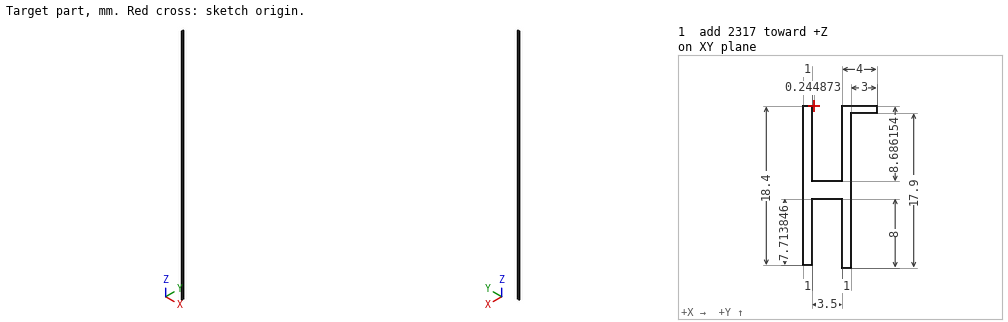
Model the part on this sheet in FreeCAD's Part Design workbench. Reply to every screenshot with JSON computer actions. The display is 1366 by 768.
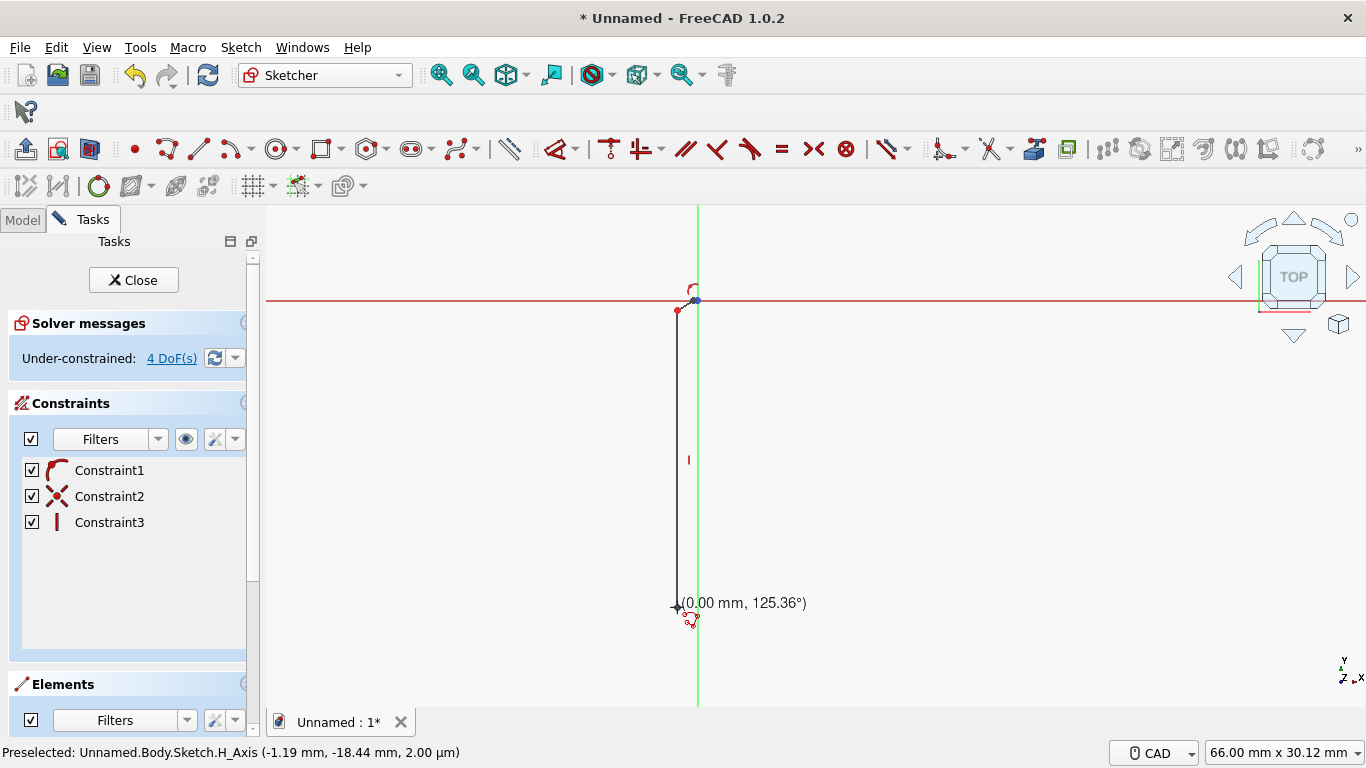
{"action": "scroll", "coordinate": [694, 607], "scroll_direction": "up", "scroll_amount": 7}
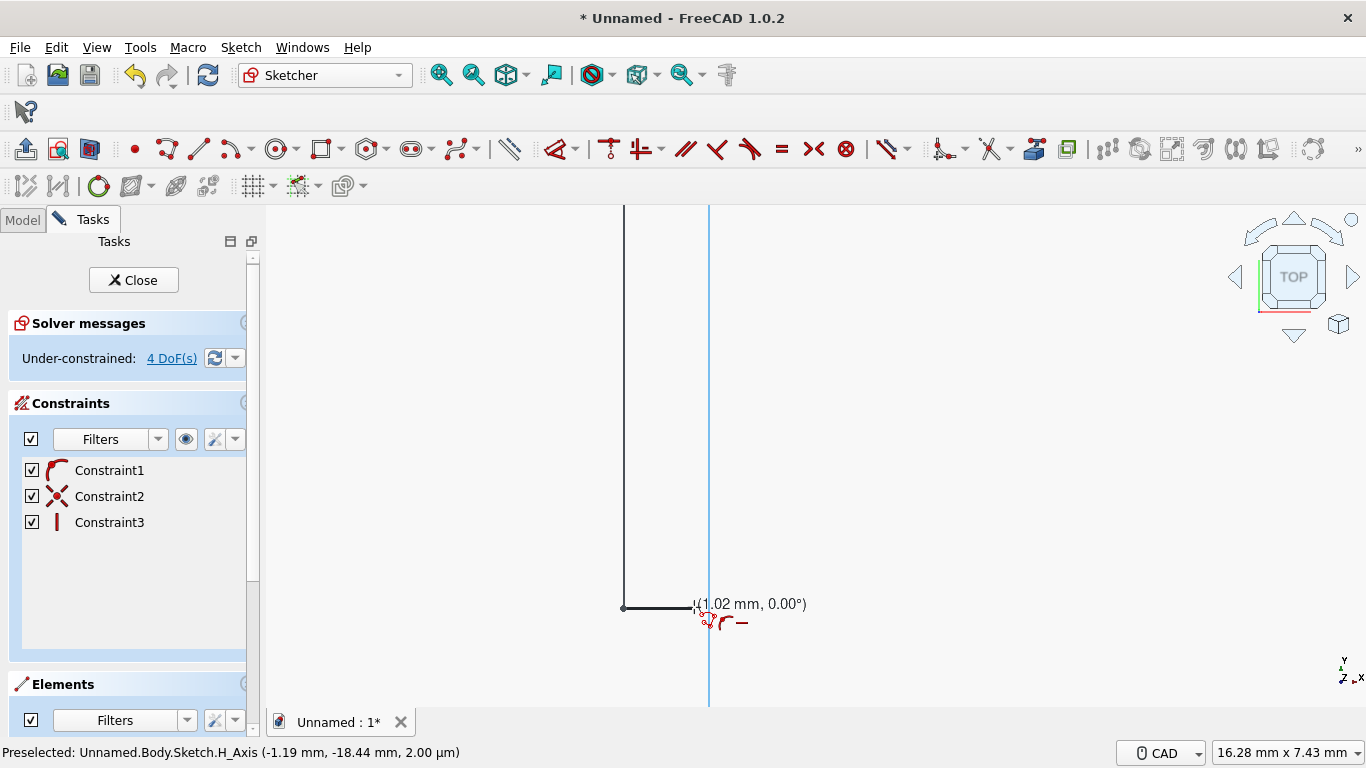
{"action": "left_click", "coordinate": [692, 605]}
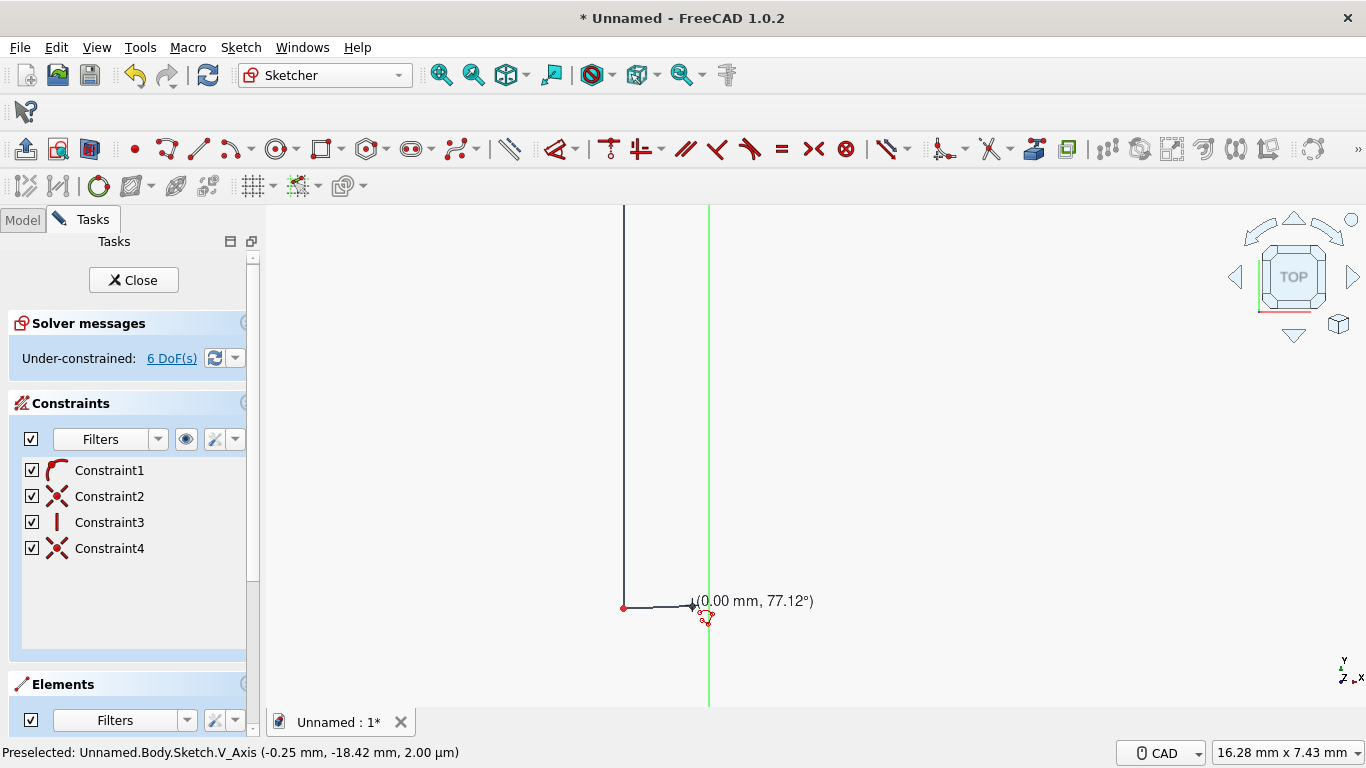
{"action": "scroll", "coordinate": [694, 607], "scroll_direction": "down", "scroll_amount": 7}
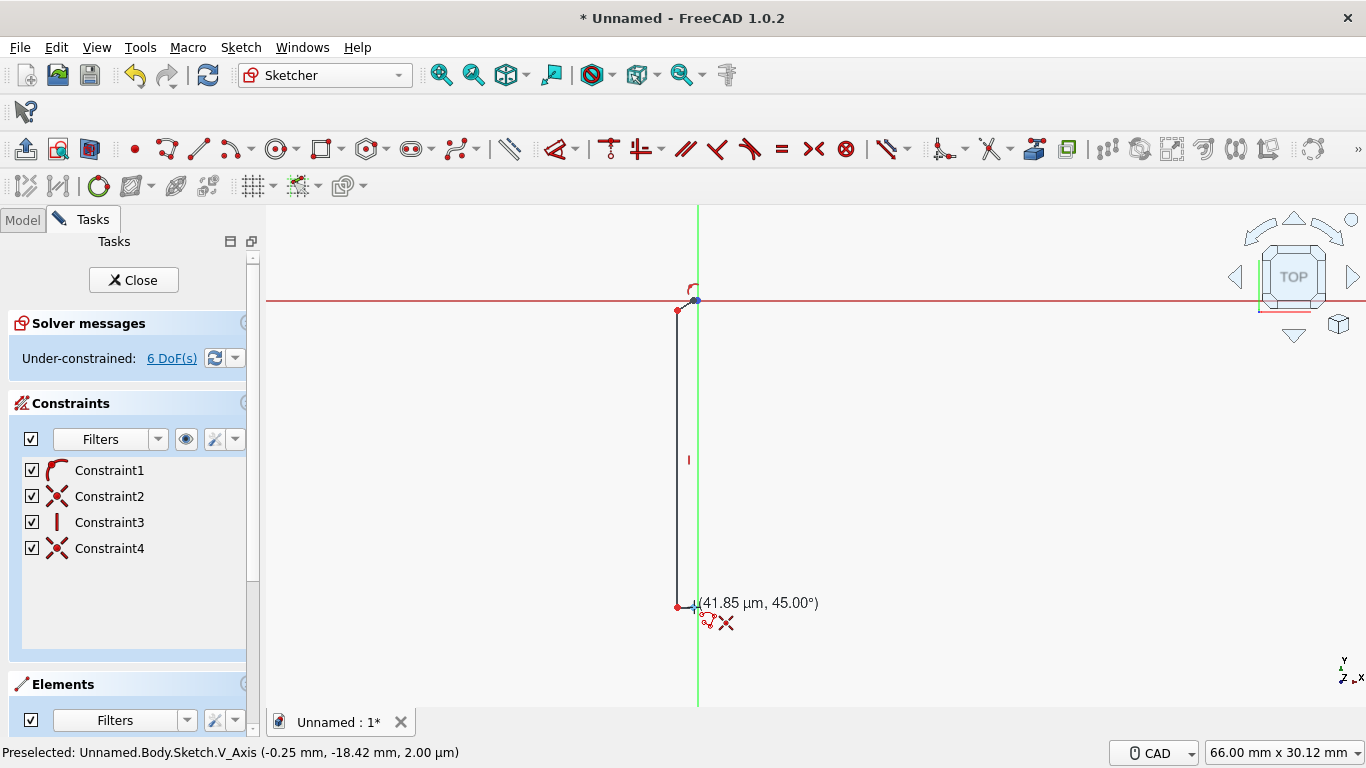
{"action": "scroll", "coordinate": [694, 479], "scroll_direction": "up", "scroll_amount": 7}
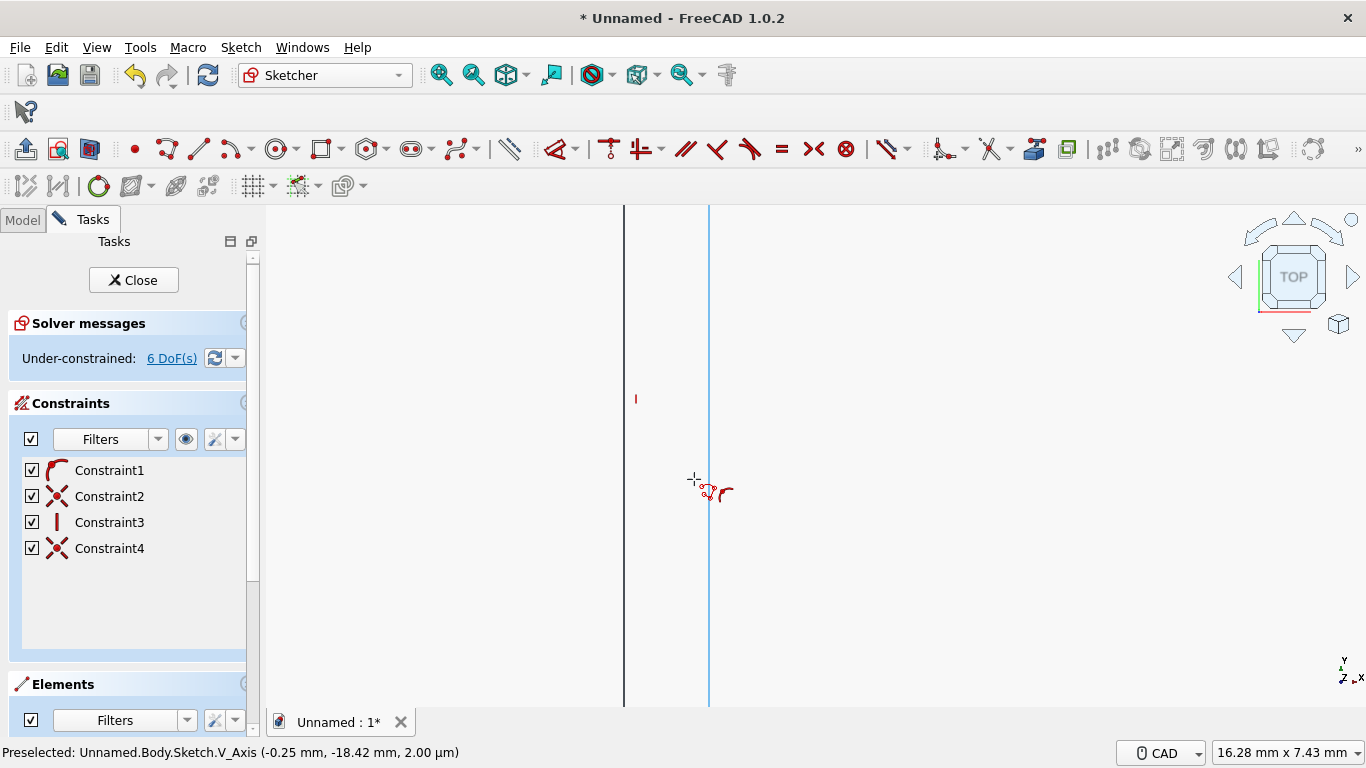
{"action": "left_click", "coordinate": [692, 476]}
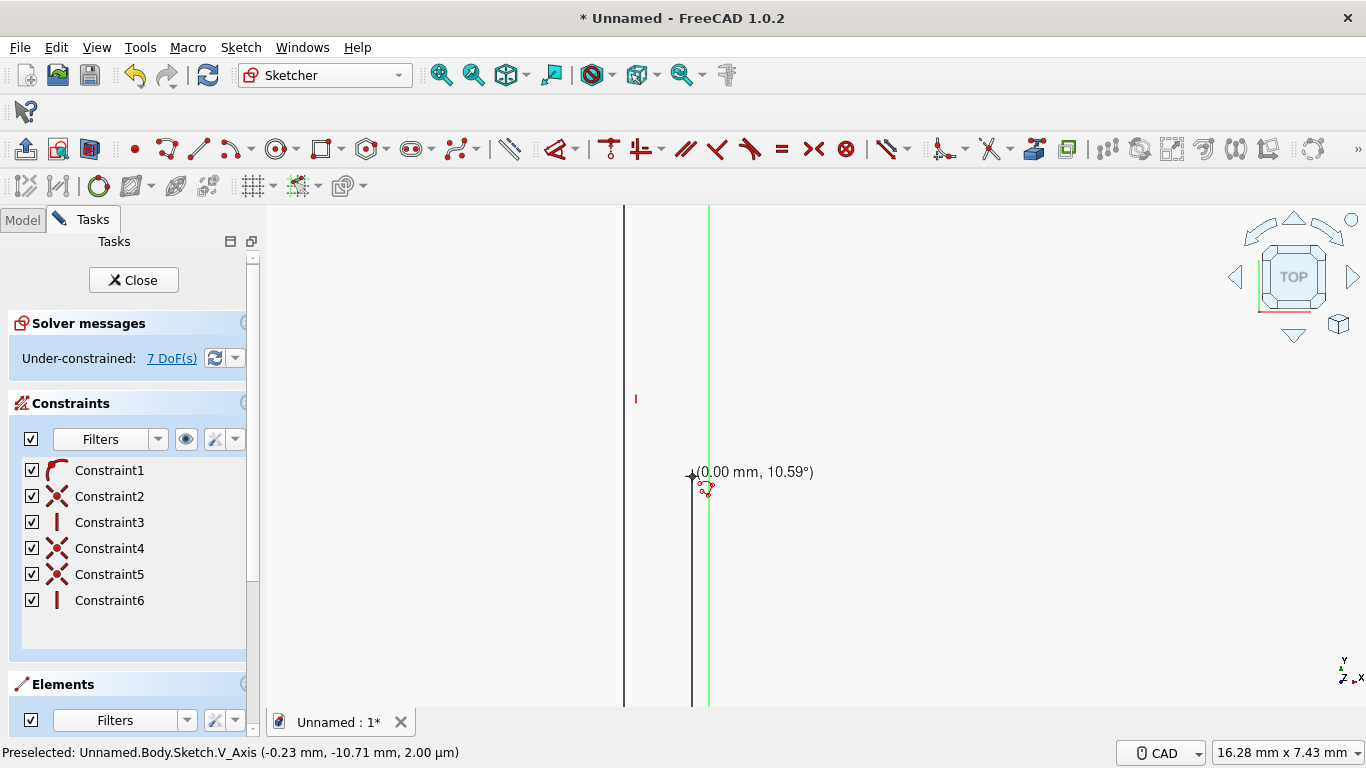
{"action": "scroll", "coordinate": [694, 479], "scroll_direction": "down", "scroll_amount": 7}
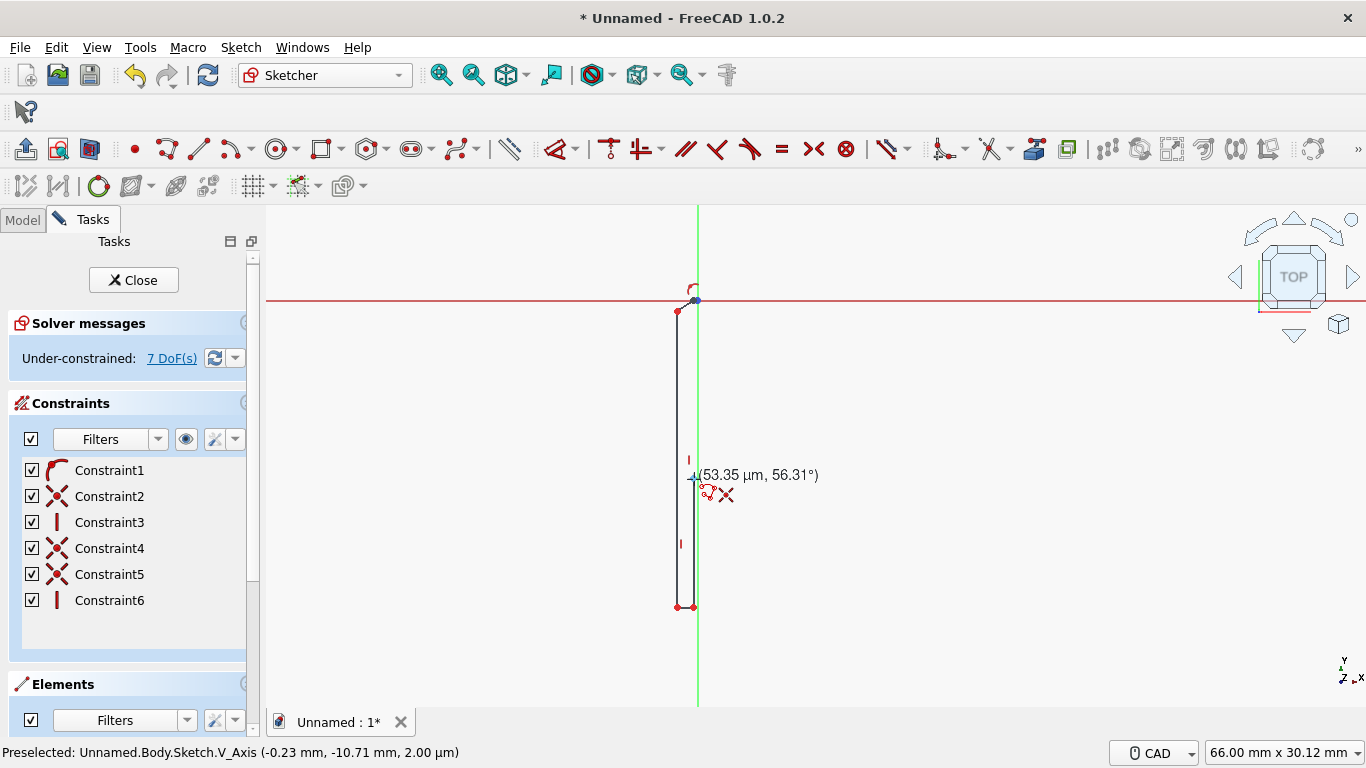
{"action": "left_click", "coordinate": [752, 479]}
{"action": "left_click", "coordinate": [752, 612]}
{"action": "left_click", "coordinate": [769, 612]}
{"action": "left_click", "coordinate": [769, 314]}
{"action": "left_click", "coordinate": [819, 314]}
{"action": "left_click", "coordinate": [819, 301]}
{"action": "left_click", "coordinate": [752, 310]}
{"action": "left_click", "coordinate": [752, 445]}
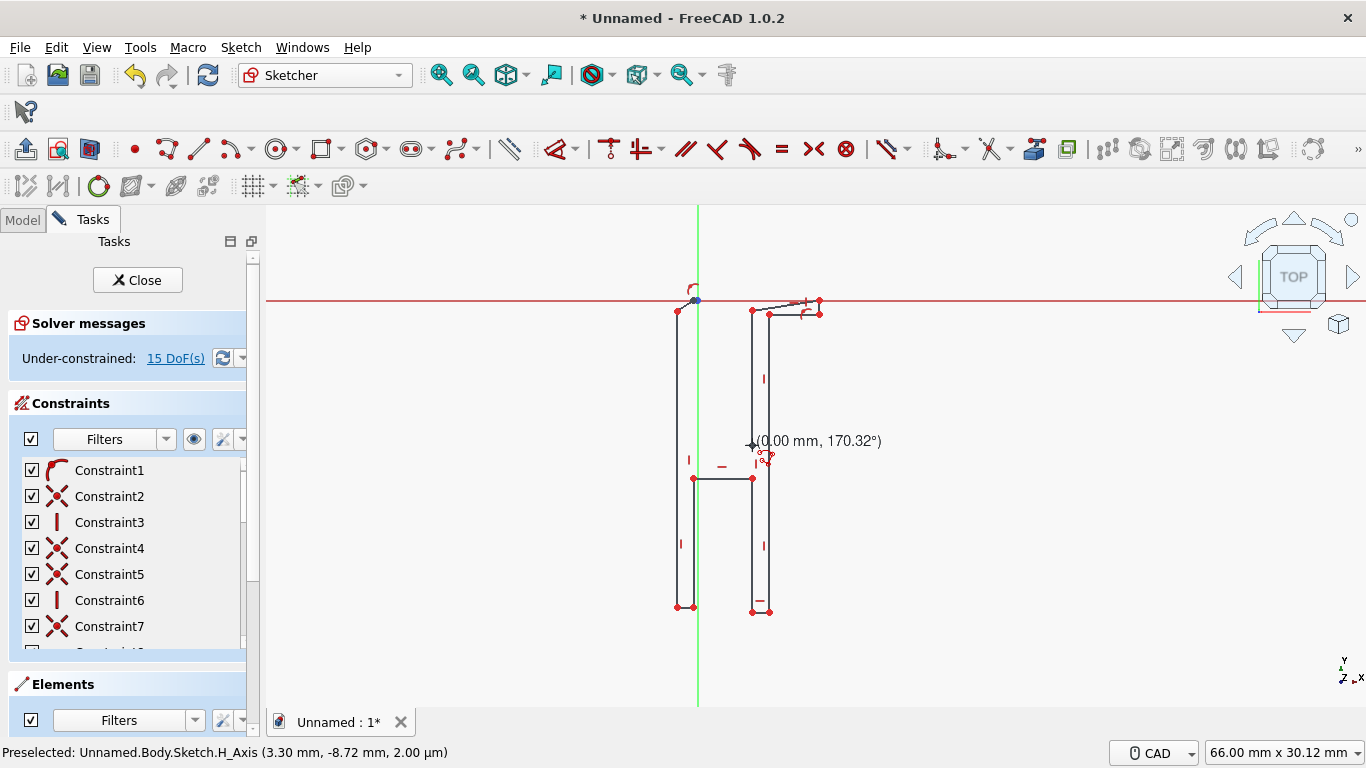
{"action": "scroll", "coordinate": [694, 445], "scroll_direction": "up", "scroll_amount": 7}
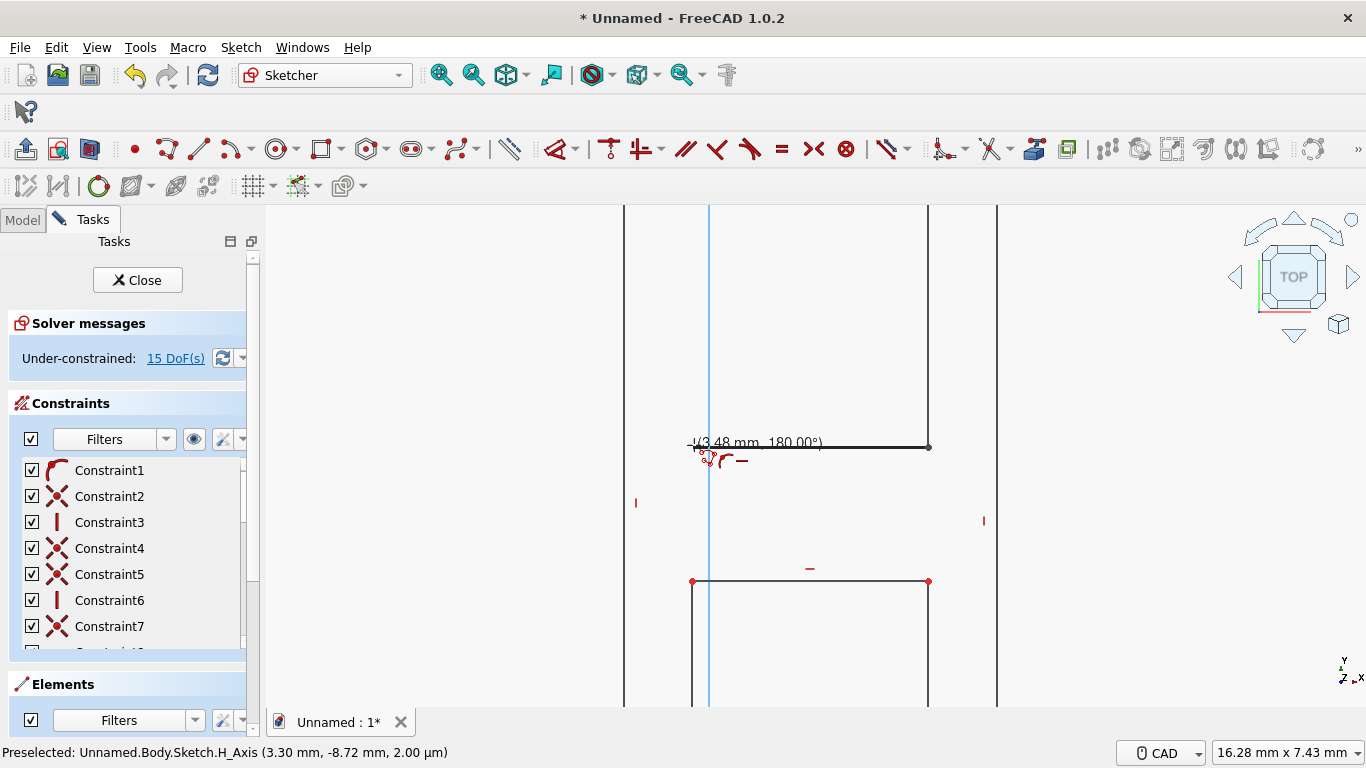
{"action": "left_click", "coordinate": [692, 444]}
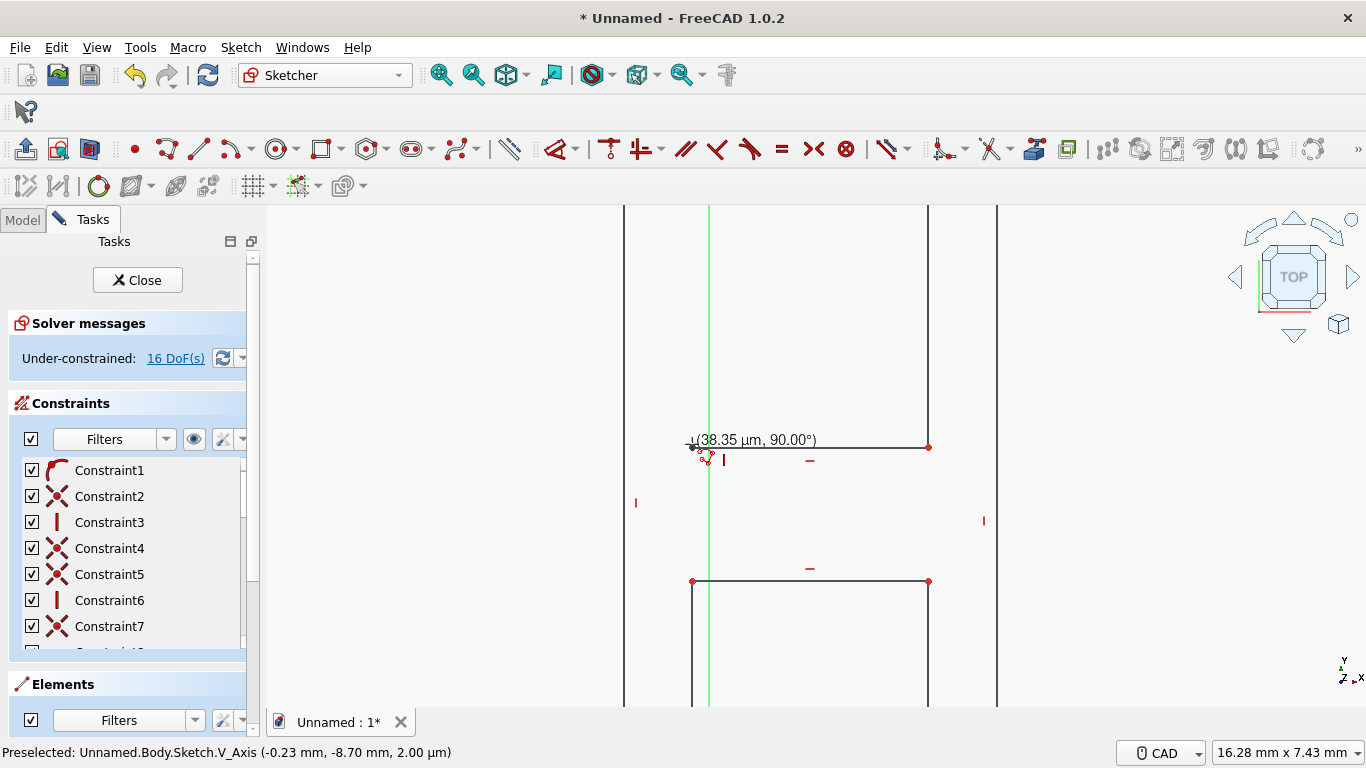
{"action": "scroll", "coordinate": [694, 445], "scroll_direction": "down", "scroll_amount": 7}